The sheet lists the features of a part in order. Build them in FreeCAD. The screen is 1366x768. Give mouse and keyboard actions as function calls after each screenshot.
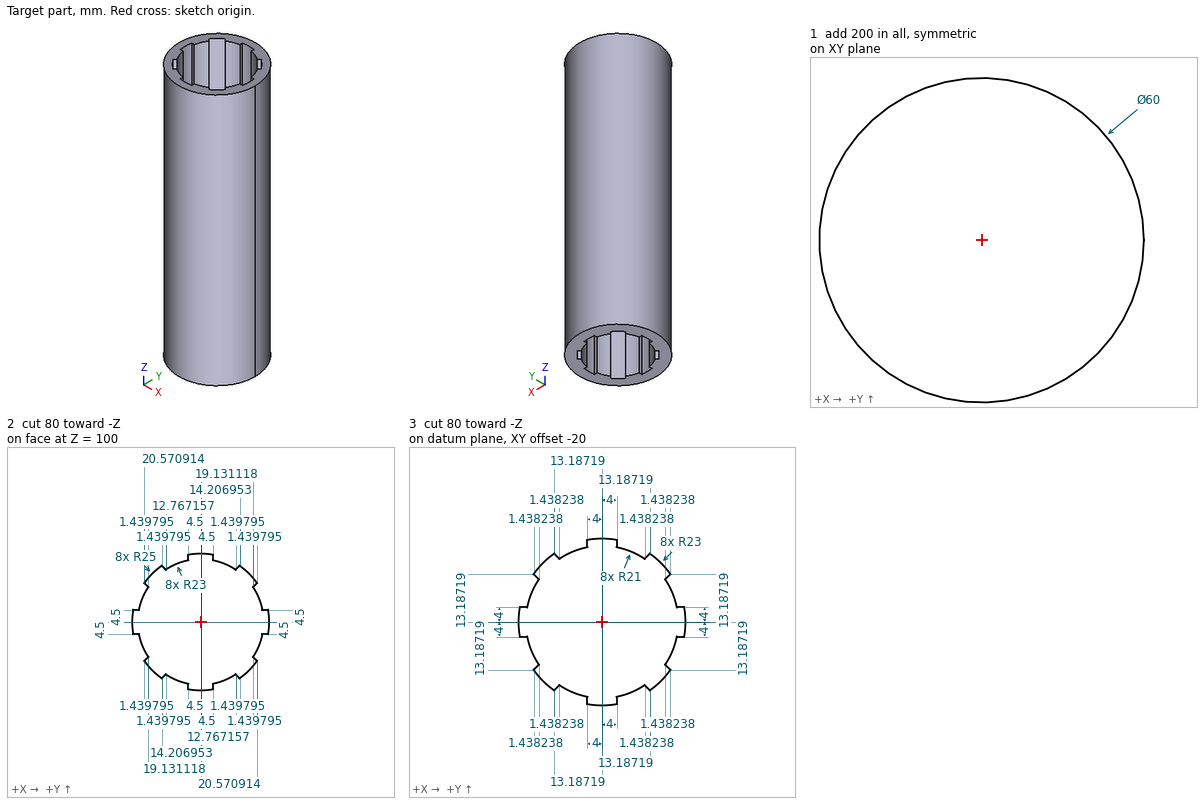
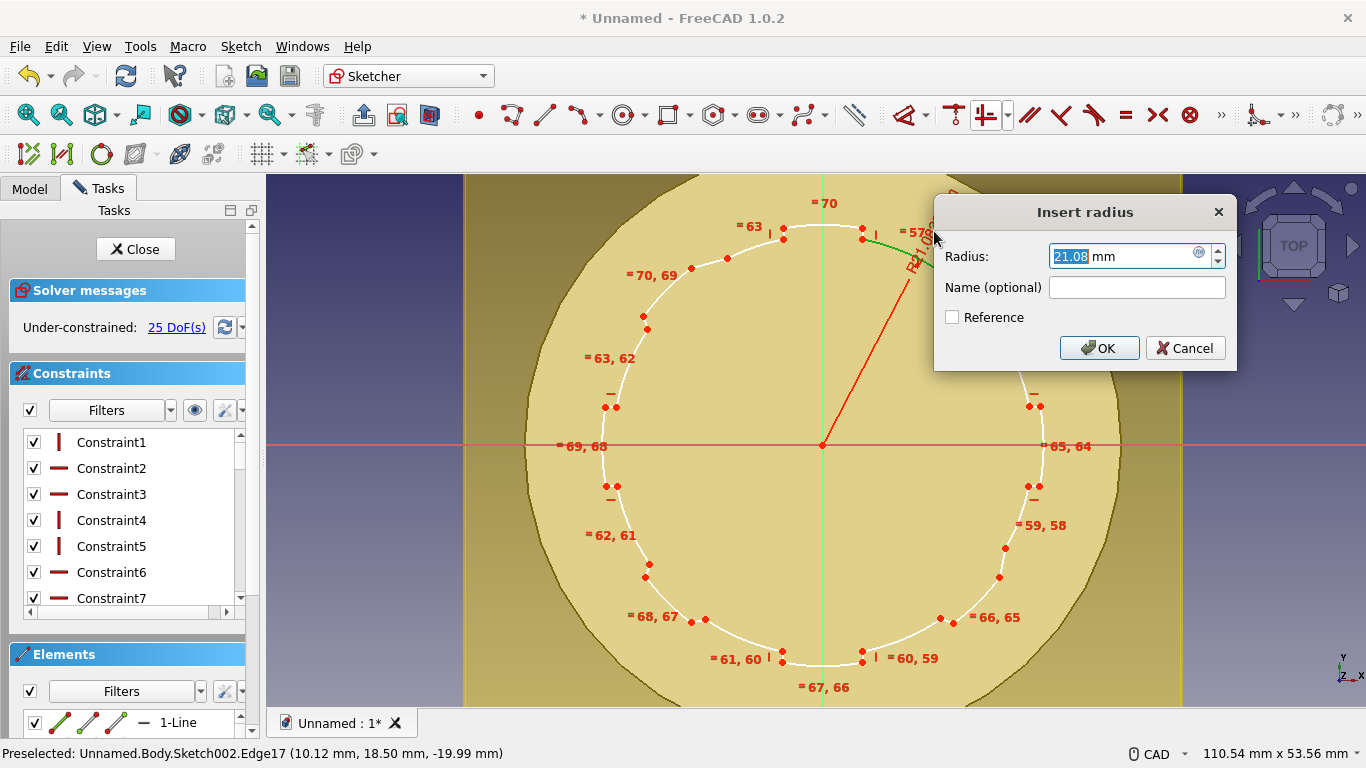
text(21)
key(Return)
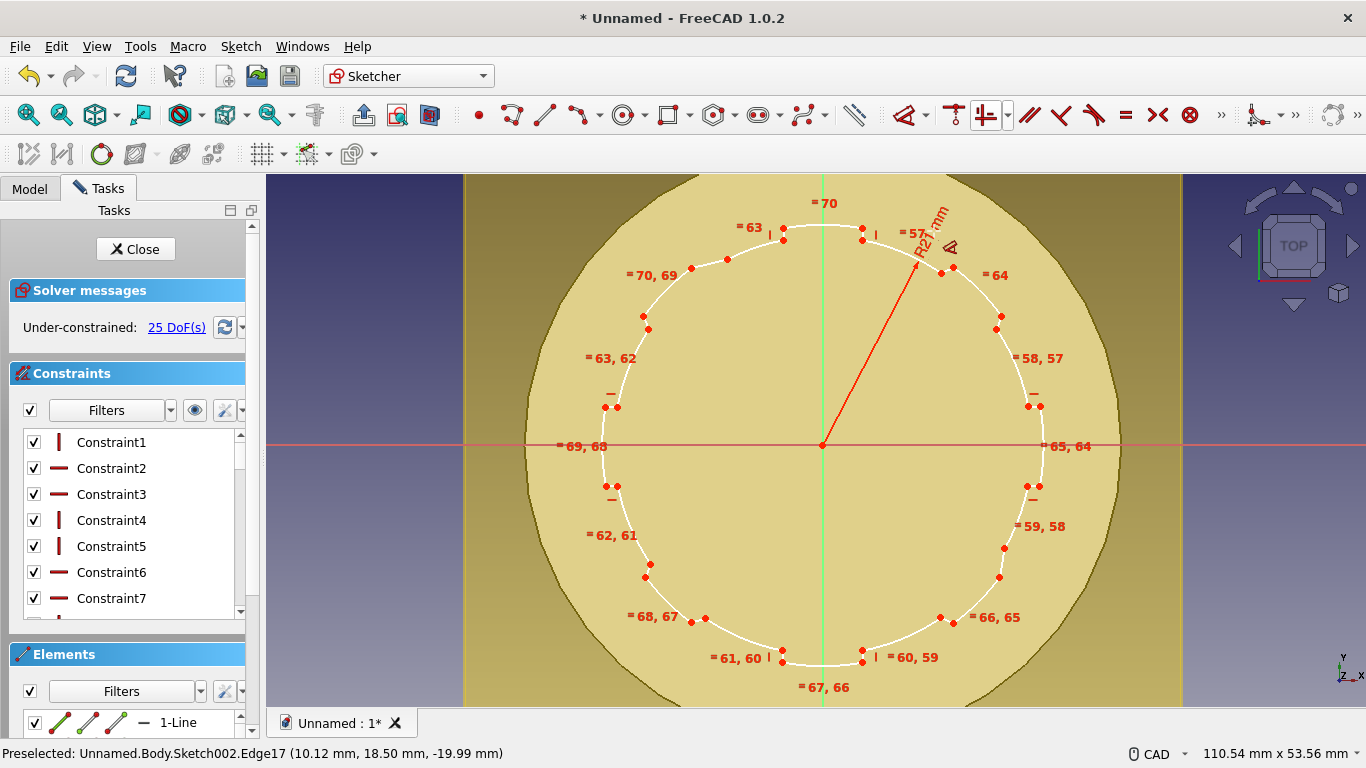
click(989, 300)
click(1013, 279)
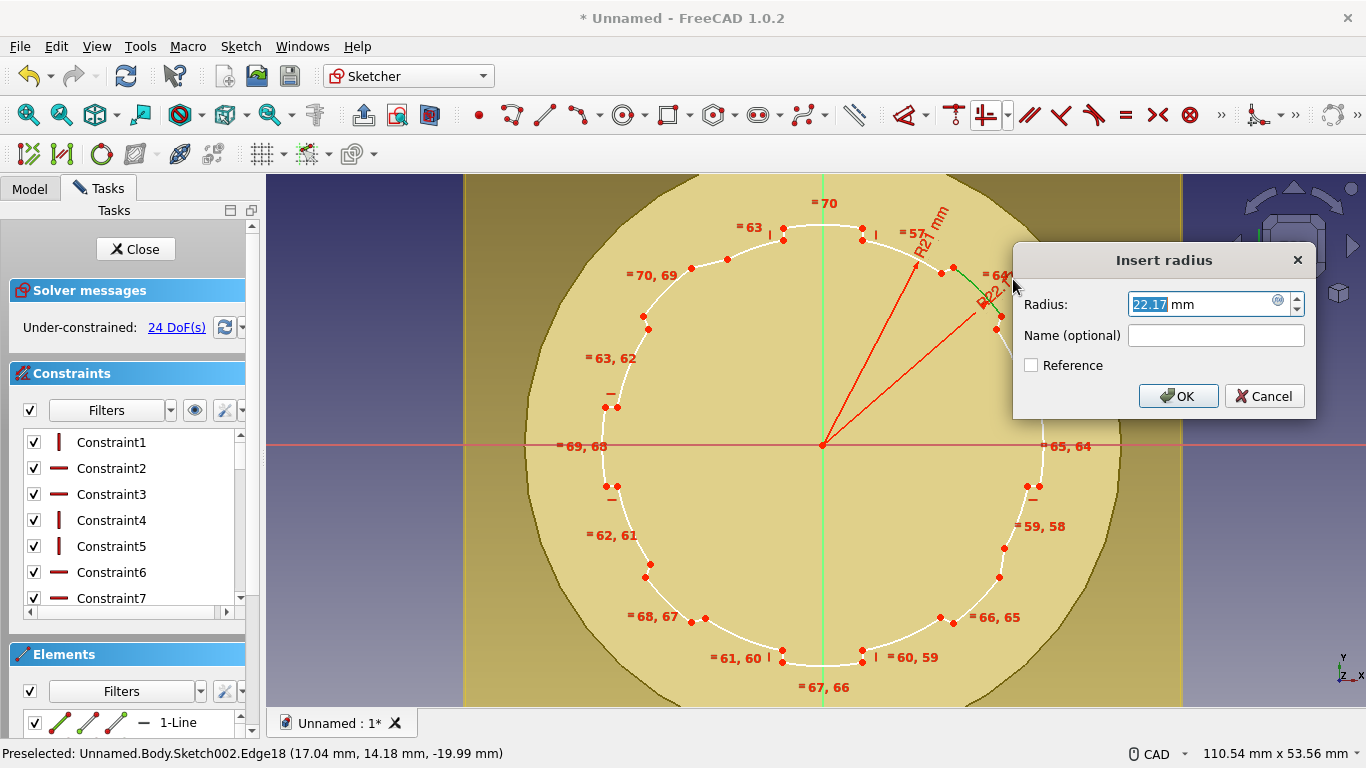
text(23)
key(Return)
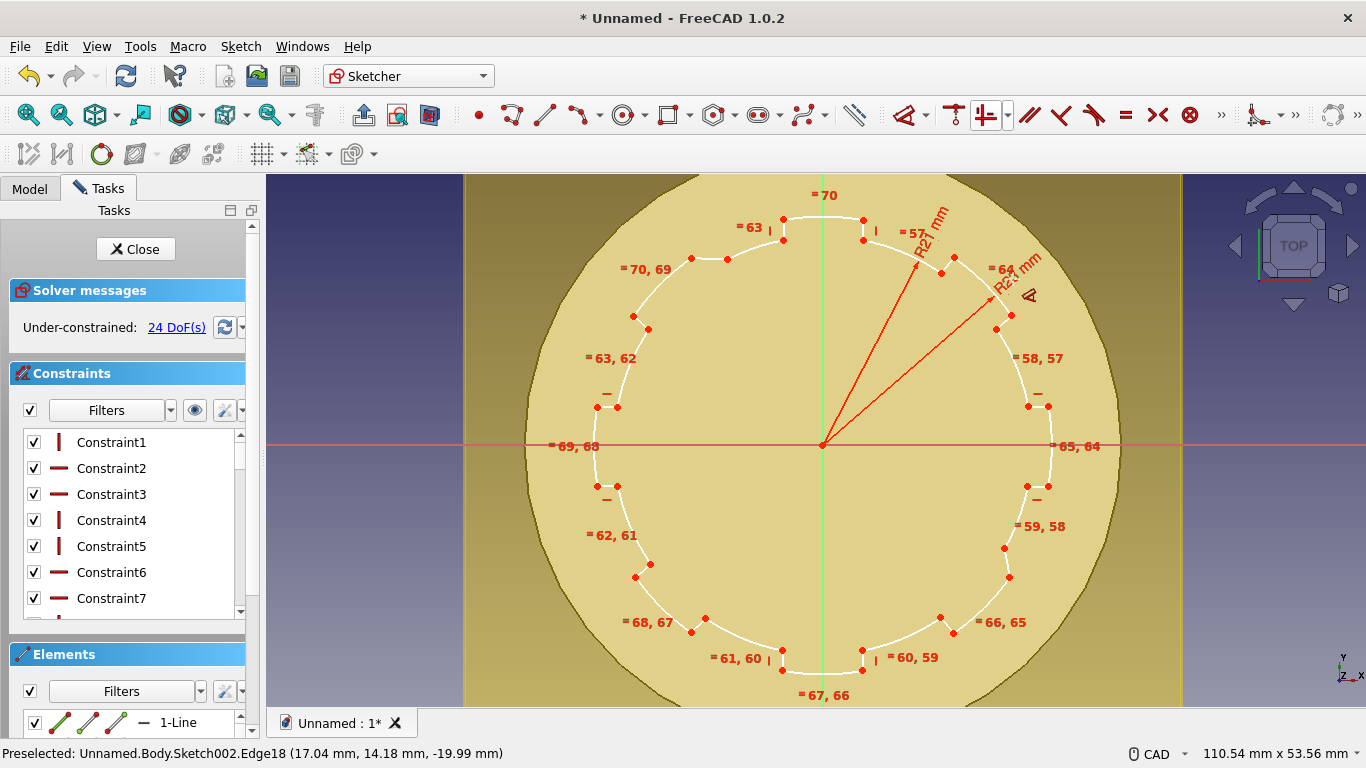
click(863, 220)
click(843, 479)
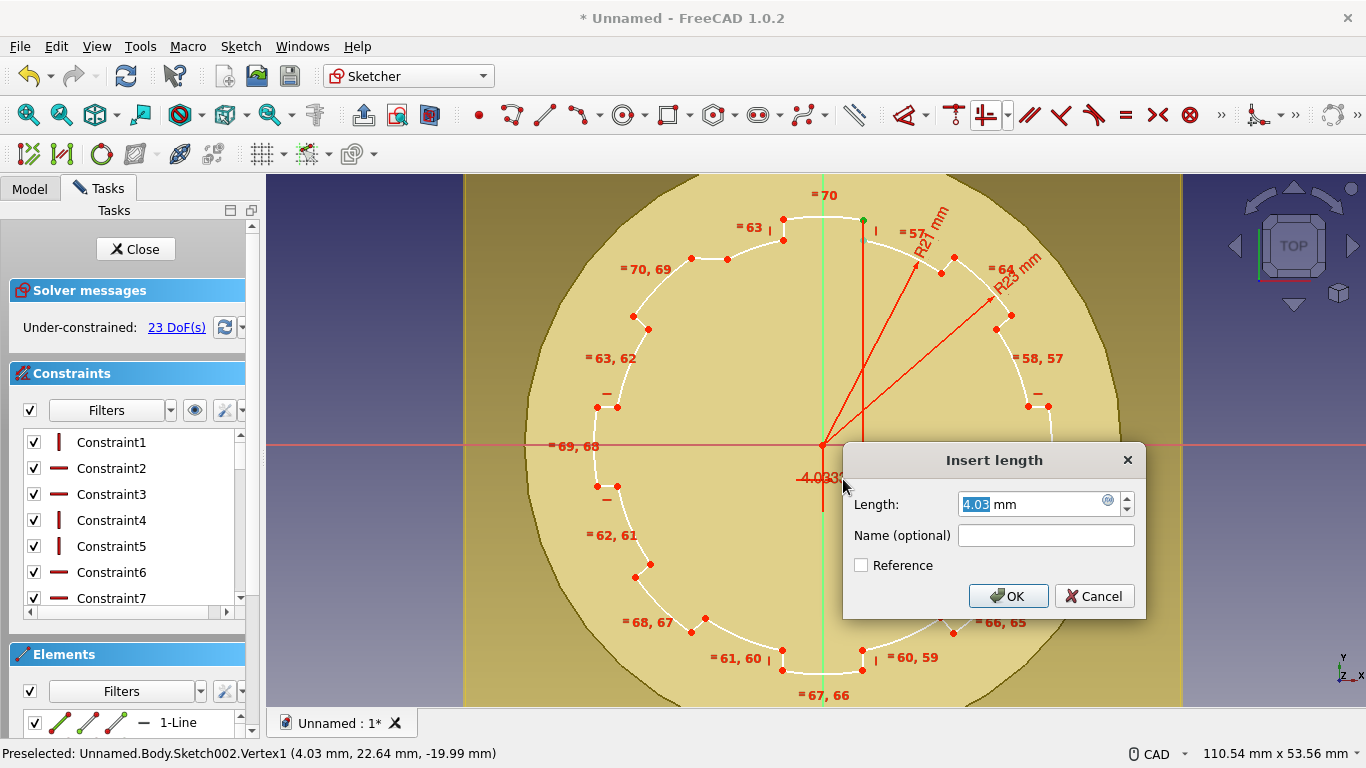
text(4)
key(Return)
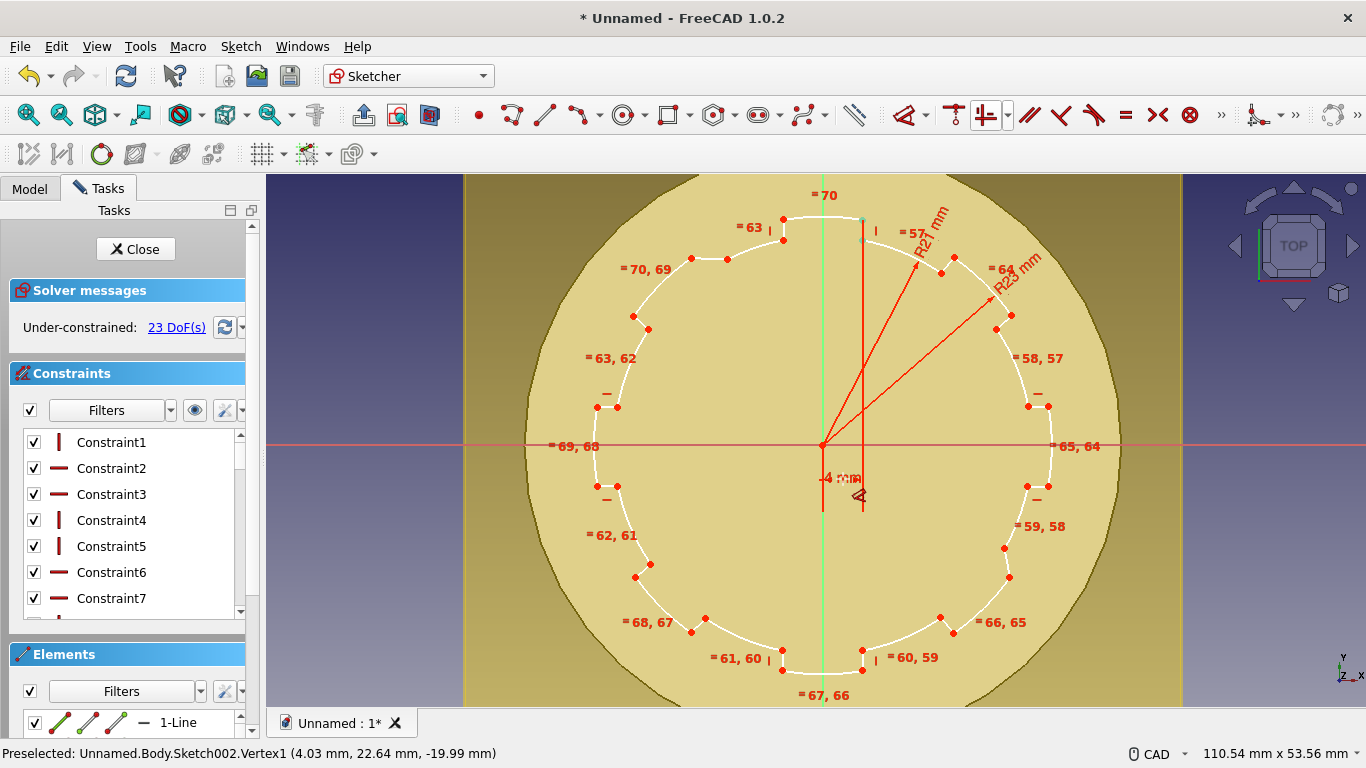
click(1028, 407)
click(789, 426)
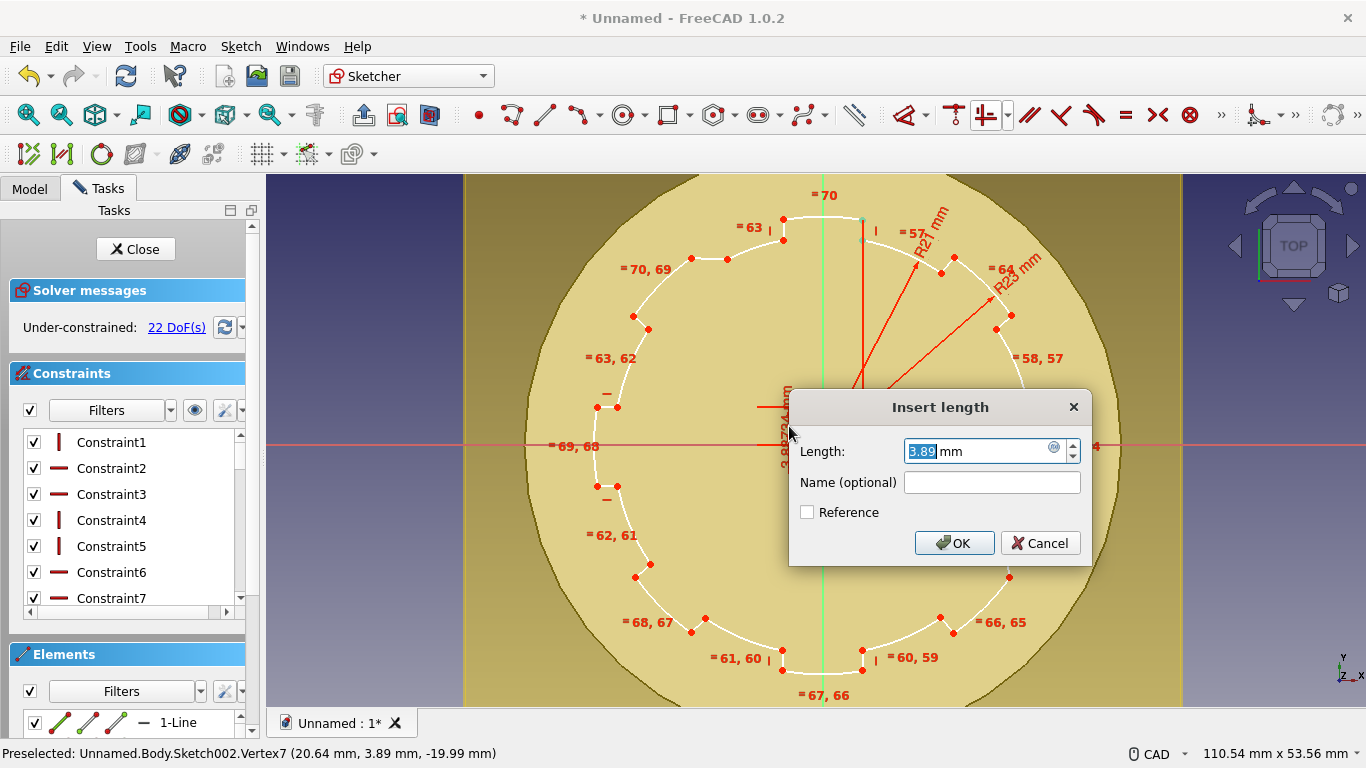
text(4)
key(Return)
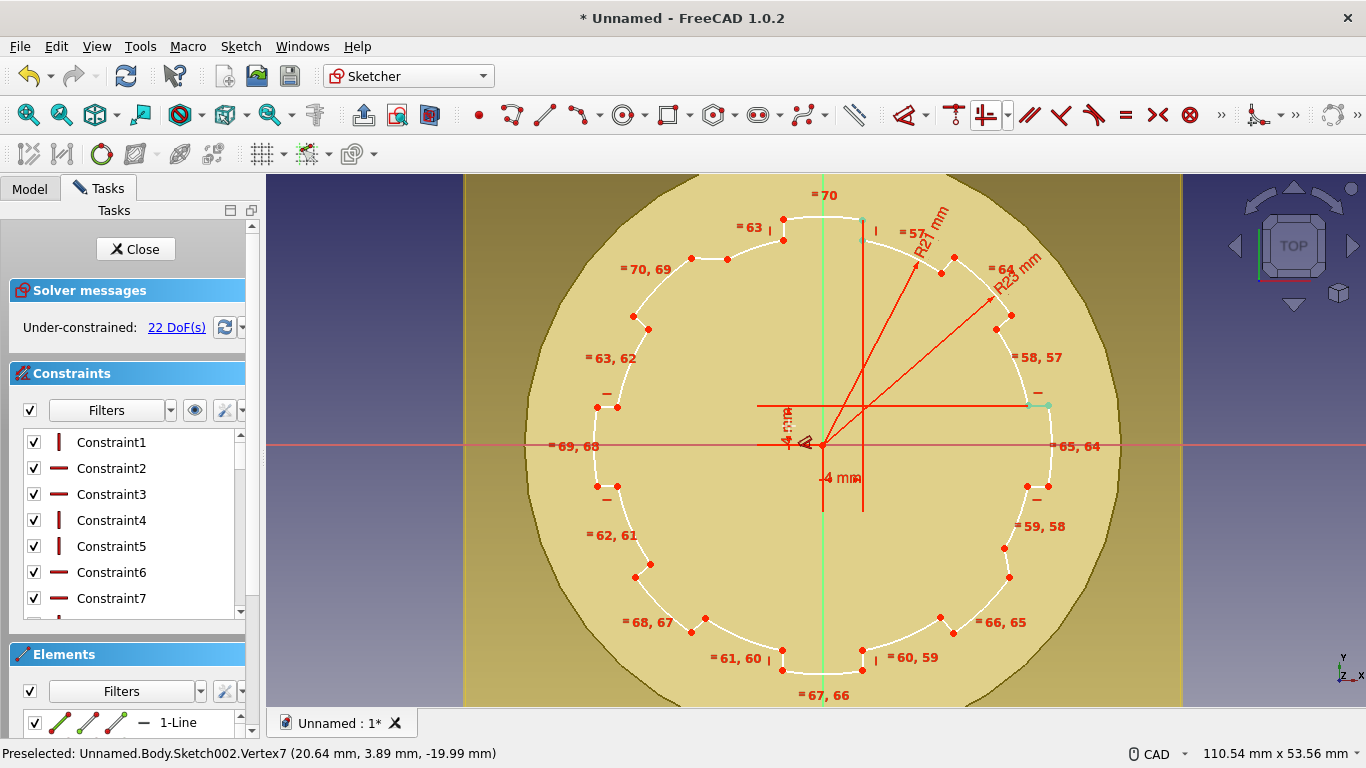
click(1048, 487)
click(1082, 466)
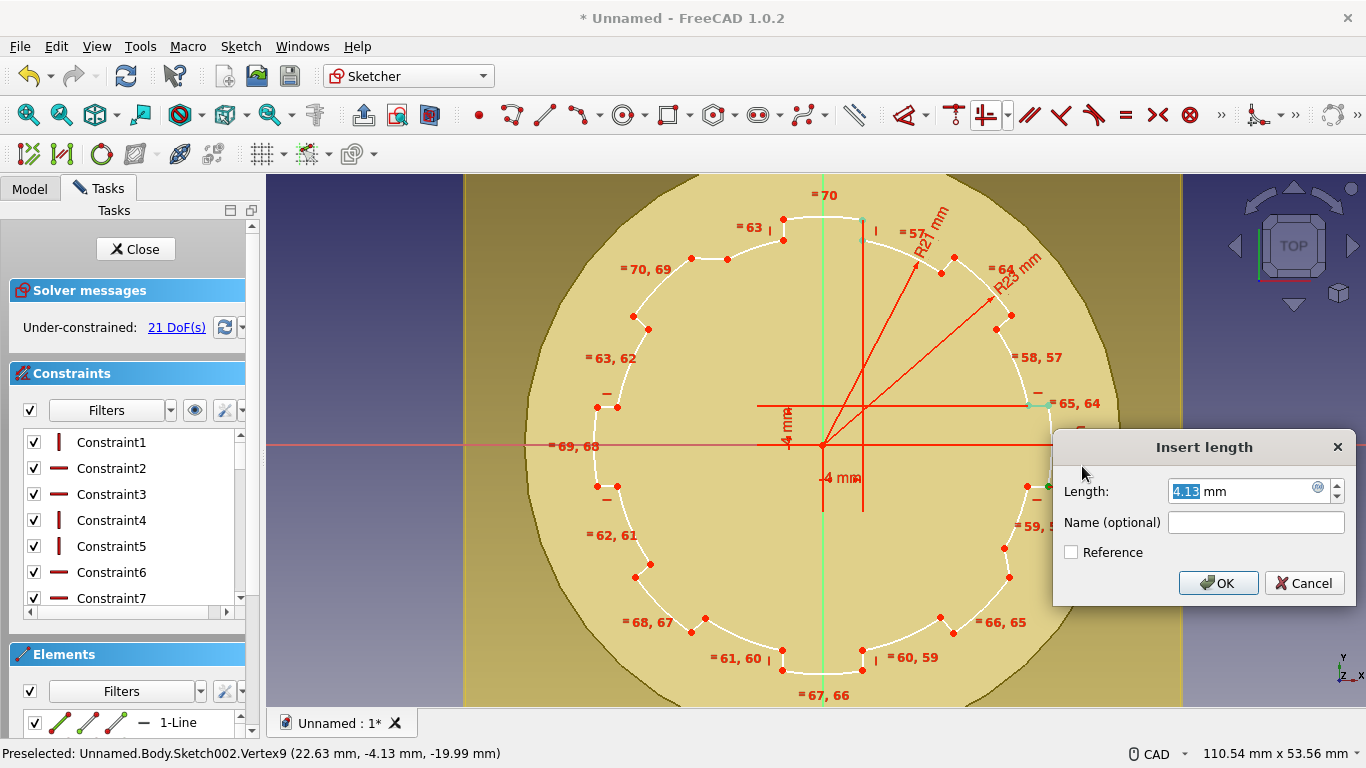
text(4)
key(Return)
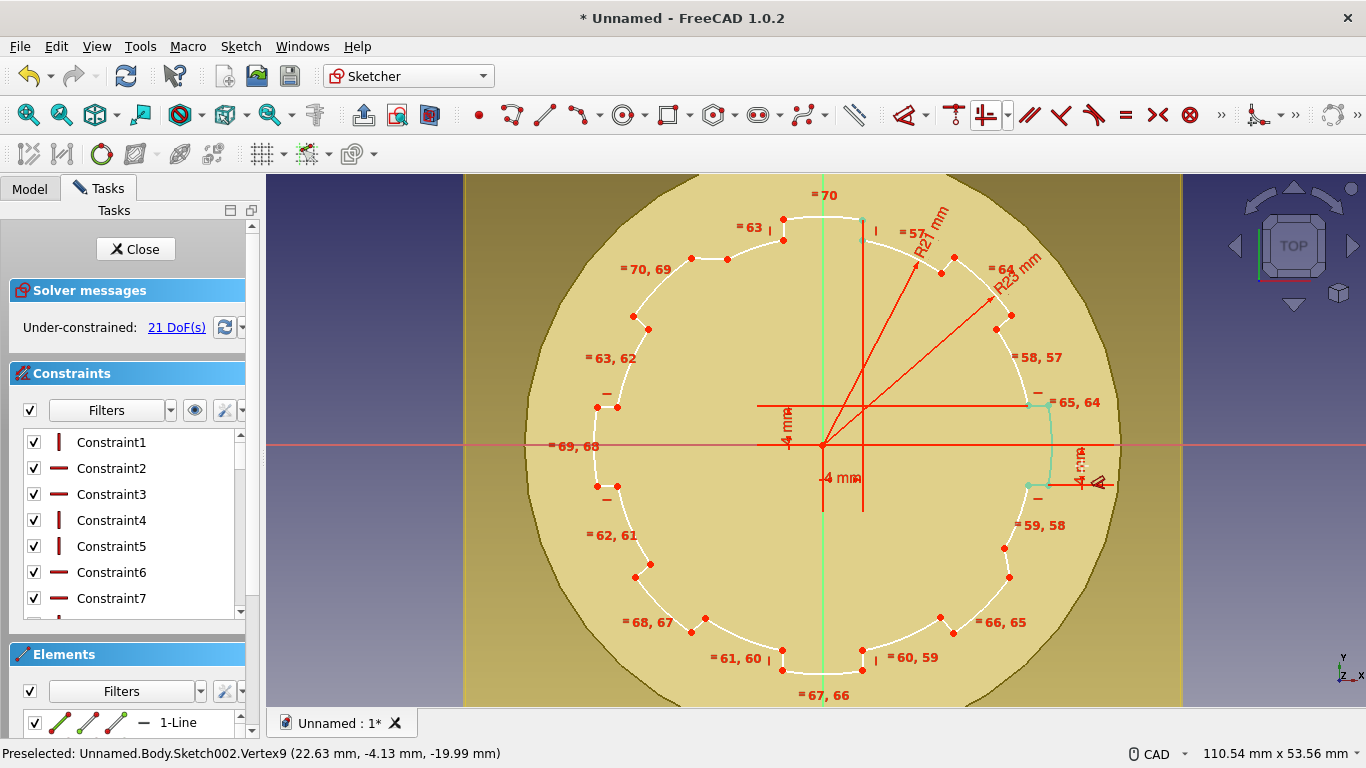
click(863, 651)
click(843, 387)